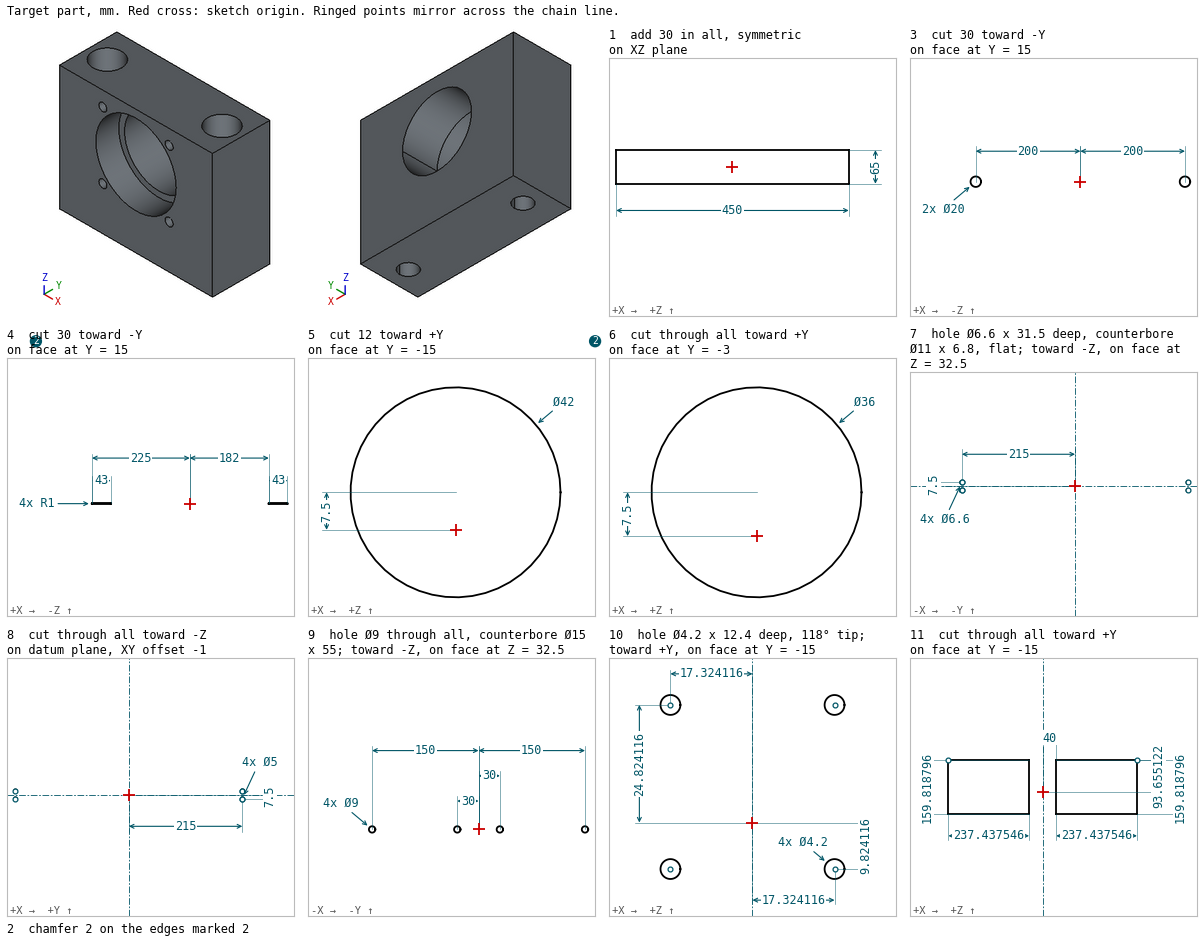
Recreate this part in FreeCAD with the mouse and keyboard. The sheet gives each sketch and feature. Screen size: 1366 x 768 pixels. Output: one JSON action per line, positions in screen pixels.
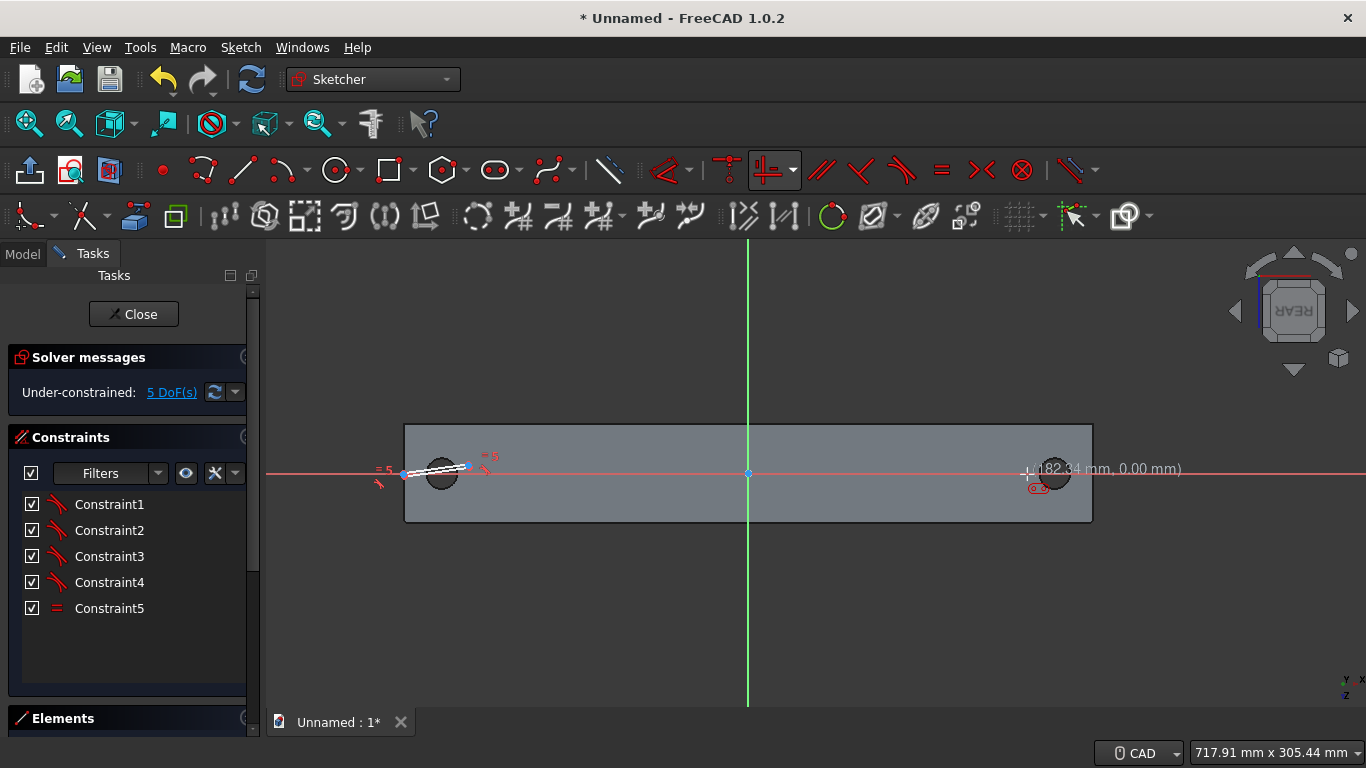
{"action": "left_click", "coordinate": [1027, 474]}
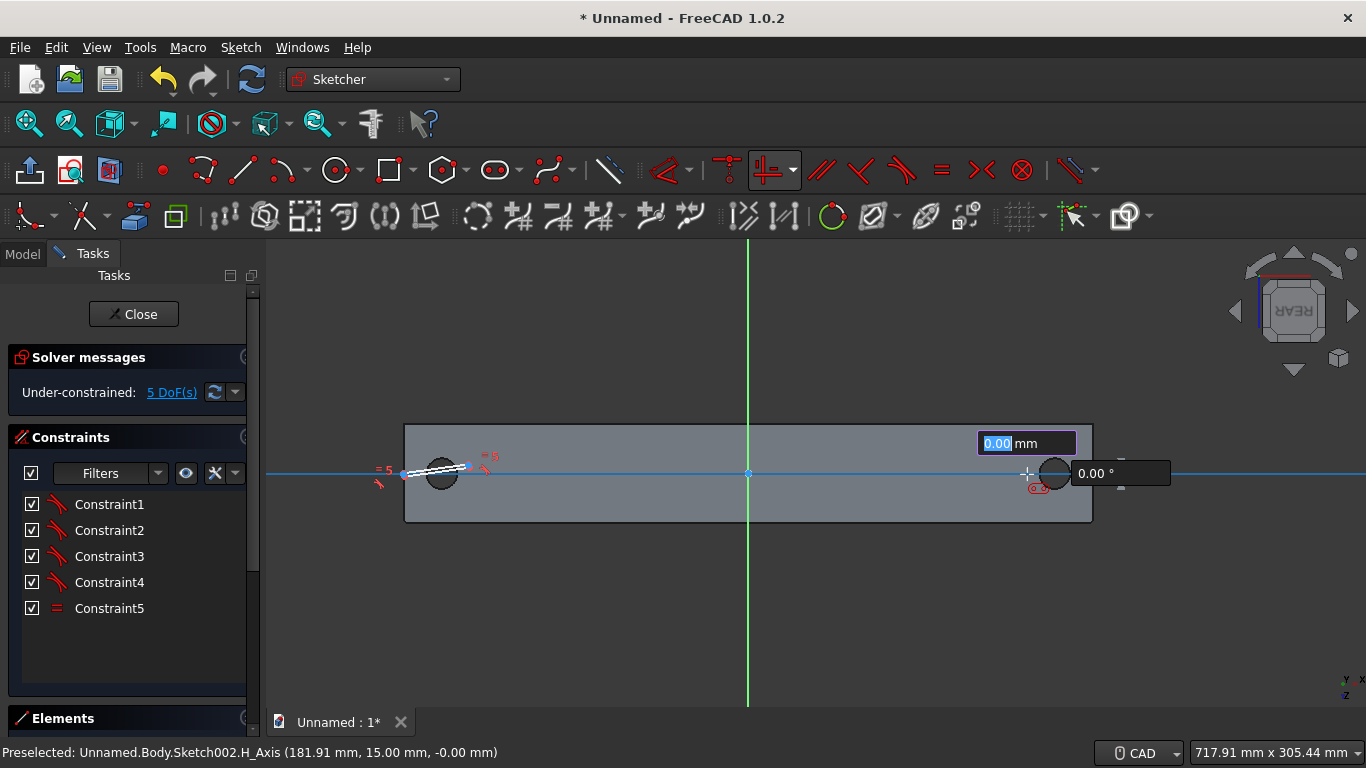
{"action": "left_click", "coordinate": [1093, 465]}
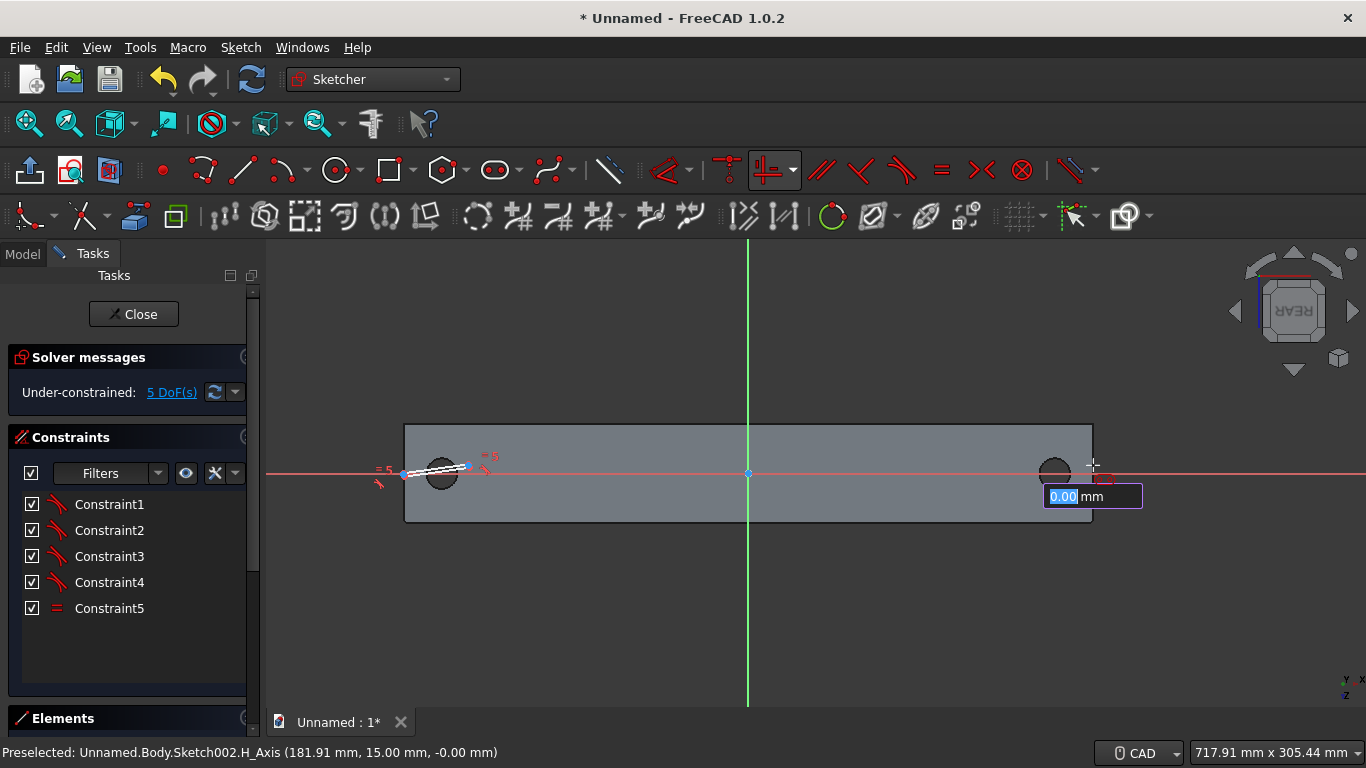
{"action": "scroll", "coordinate": [1060, 472], "scroll_direction": "up", "scroll_amount": 12}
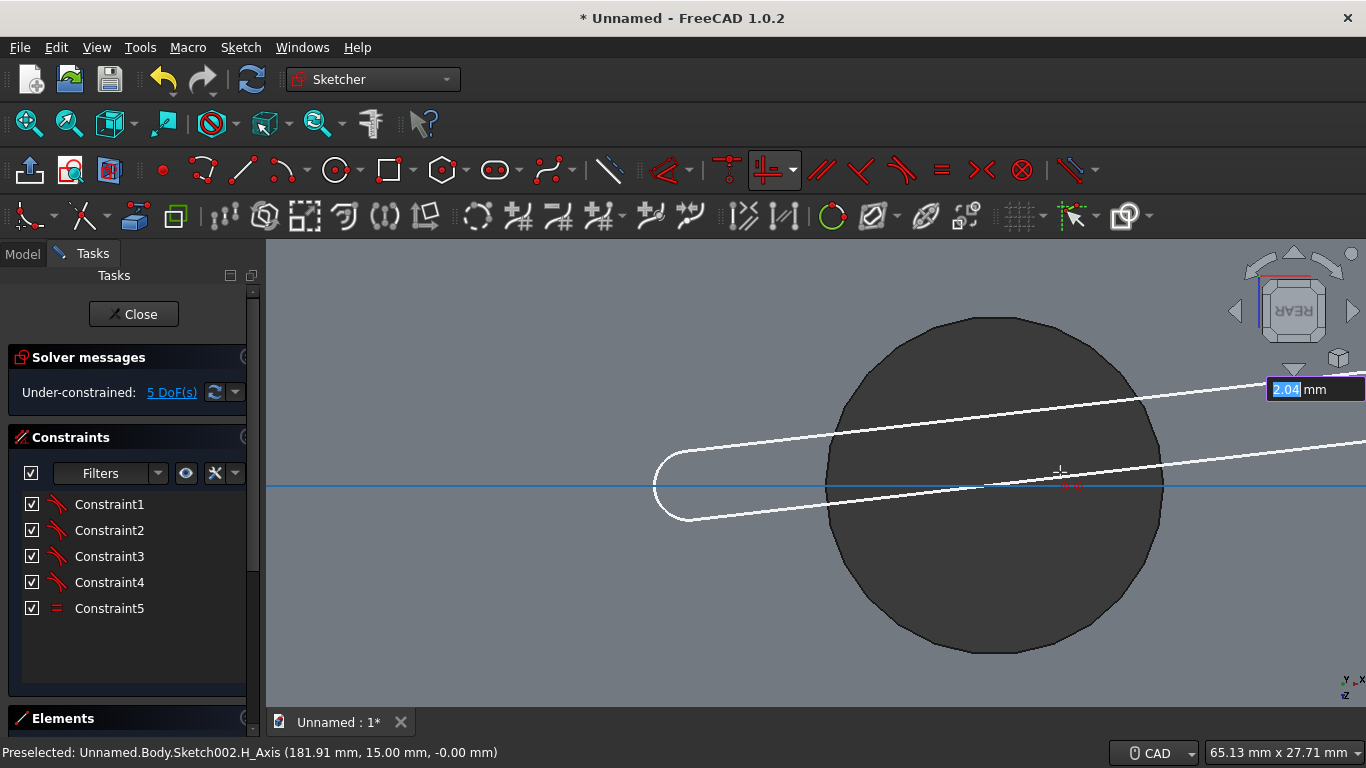
{"action": "left_click", "coordinate": [1054, 469]}
{"action": "key", "text": "Escape"}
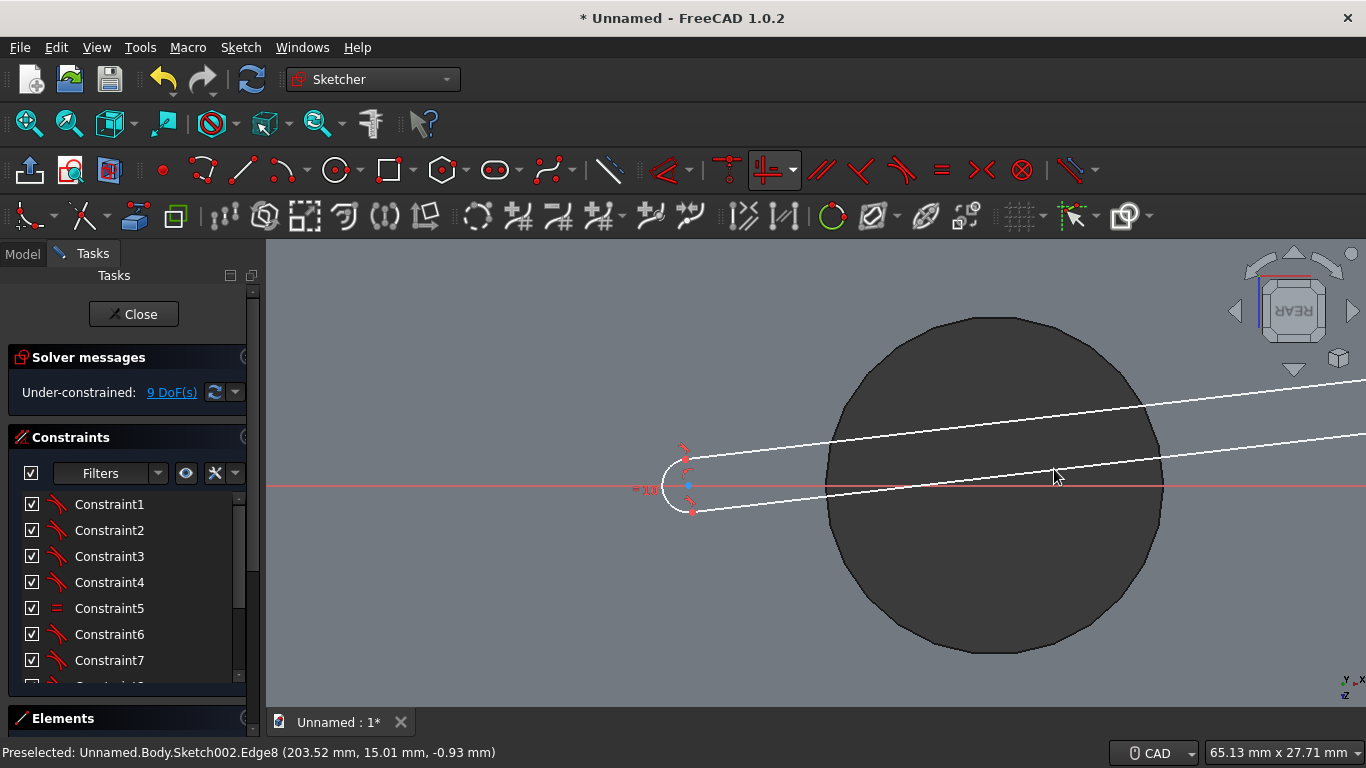
{"action": "scroll", "coordinate": [1060, 472], "scroll_direction": "down", "scroll_amount": 12}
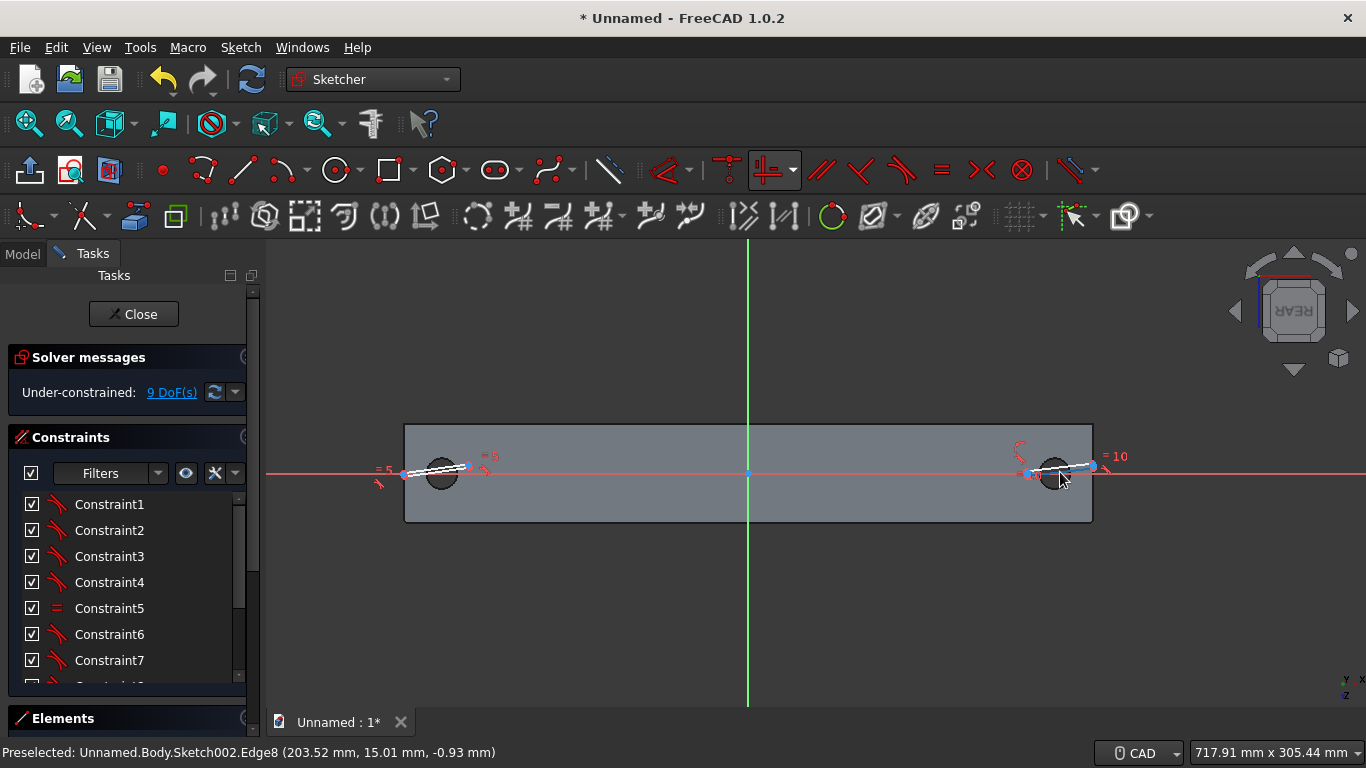
{"action": "scroll", "coordinate": [423, 471], "scroll_direction": "up", "scroll_amount": 8}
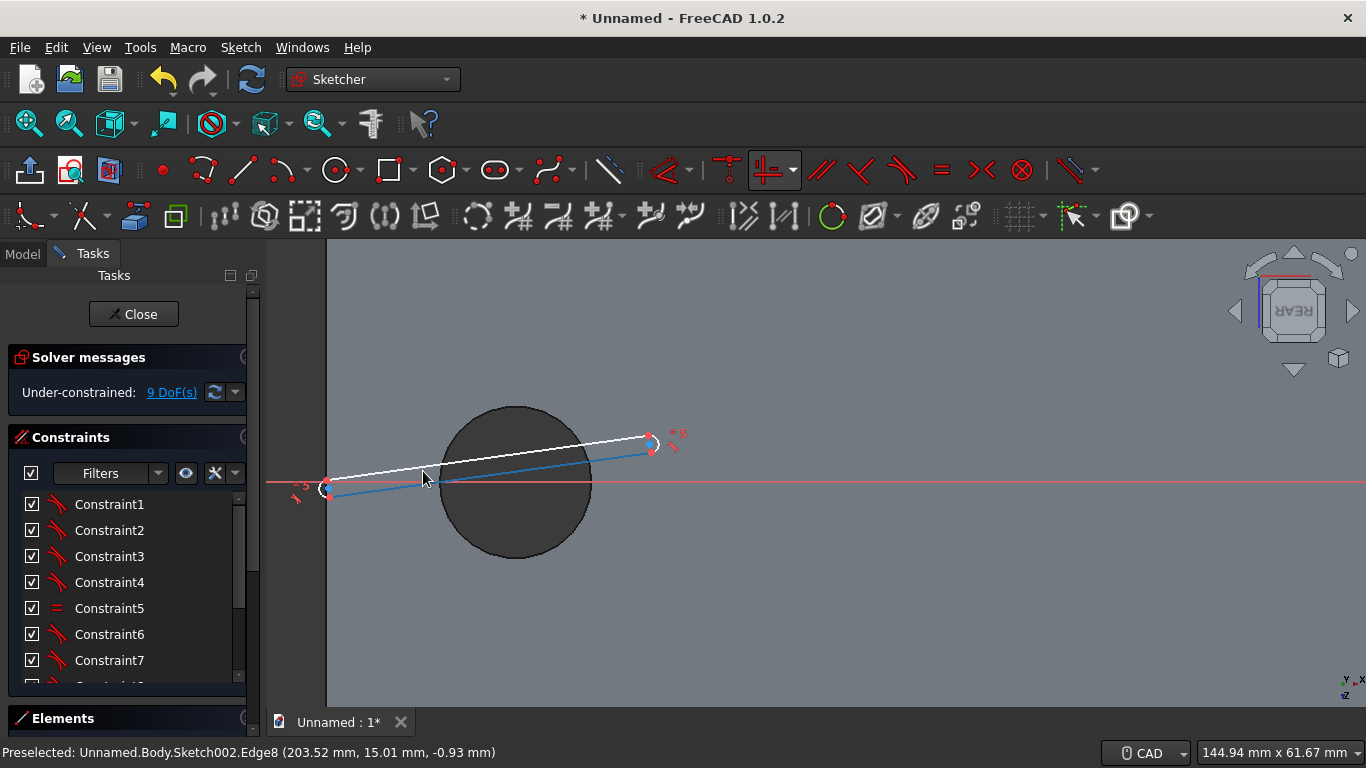
{"action": "left_click", "coordinate": [423, 467]}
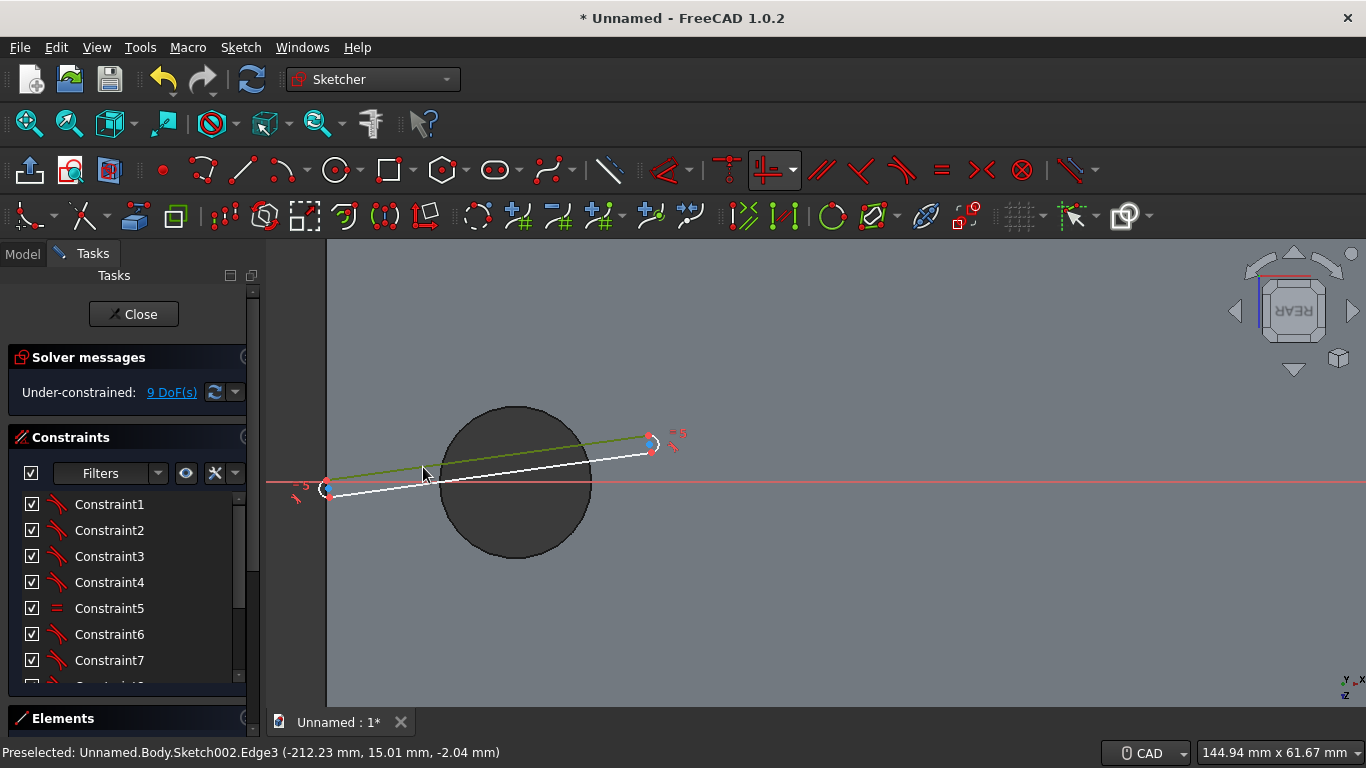
{"action": "key", "text": "h"}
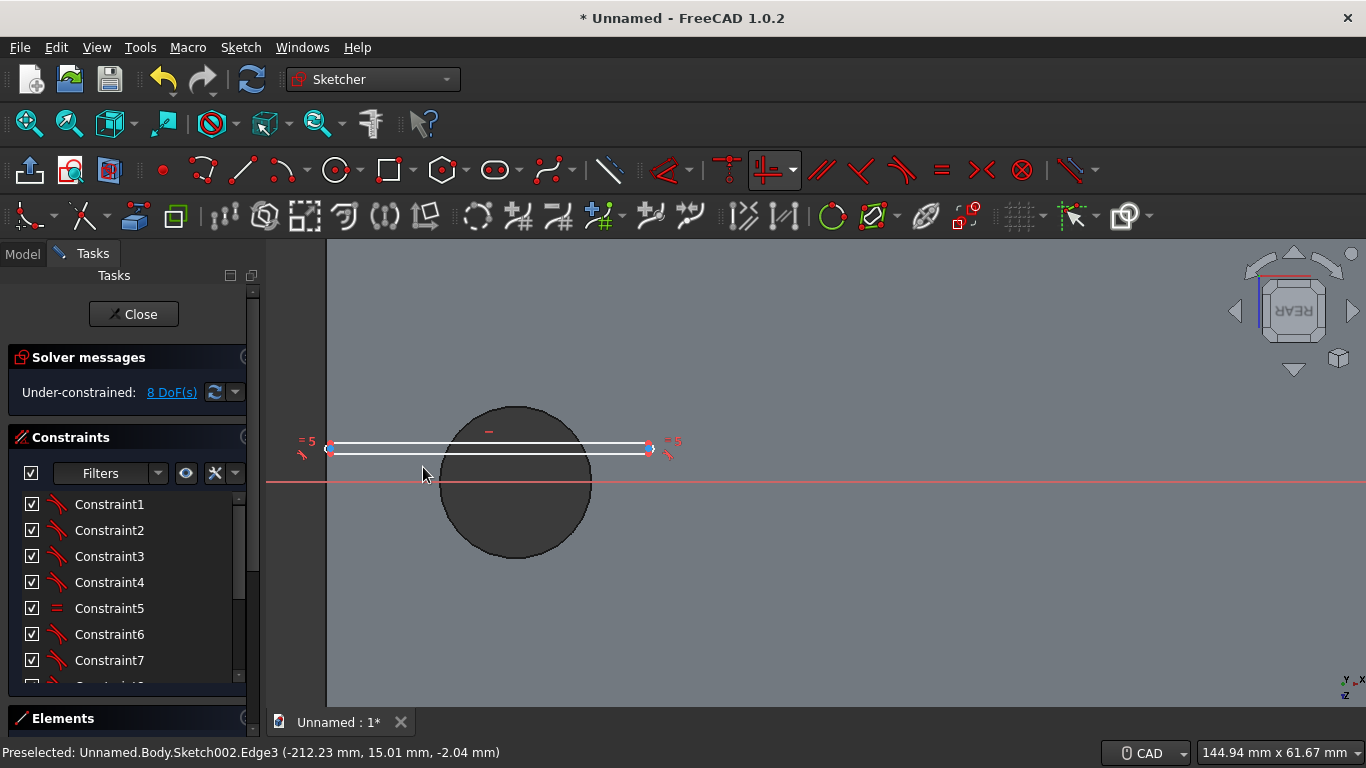
{"action": "scroll", "coordinate": [422, 471], "scroll_direction": "down", "scroll_amount": 8}